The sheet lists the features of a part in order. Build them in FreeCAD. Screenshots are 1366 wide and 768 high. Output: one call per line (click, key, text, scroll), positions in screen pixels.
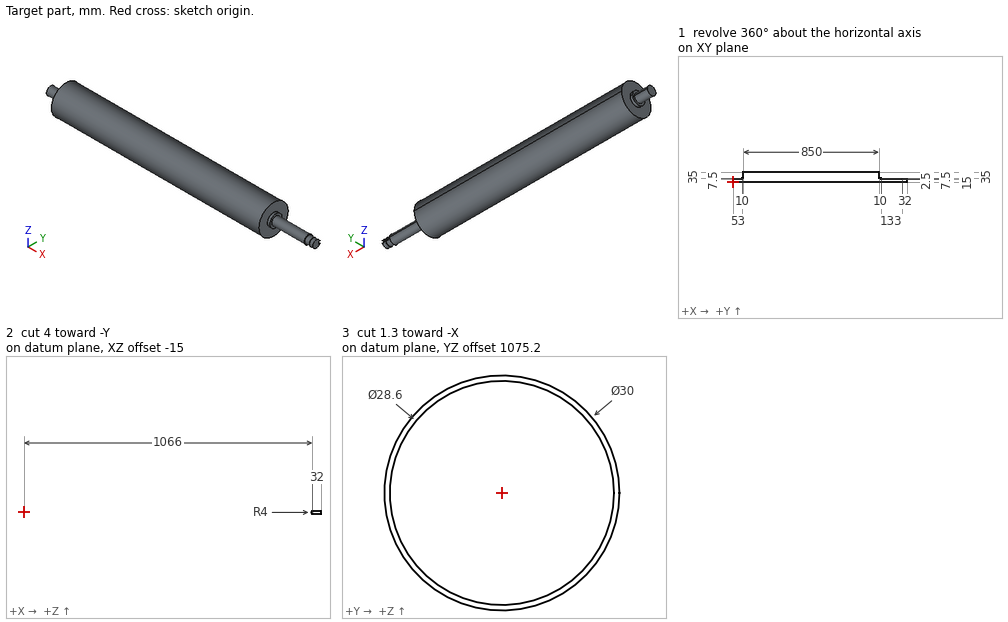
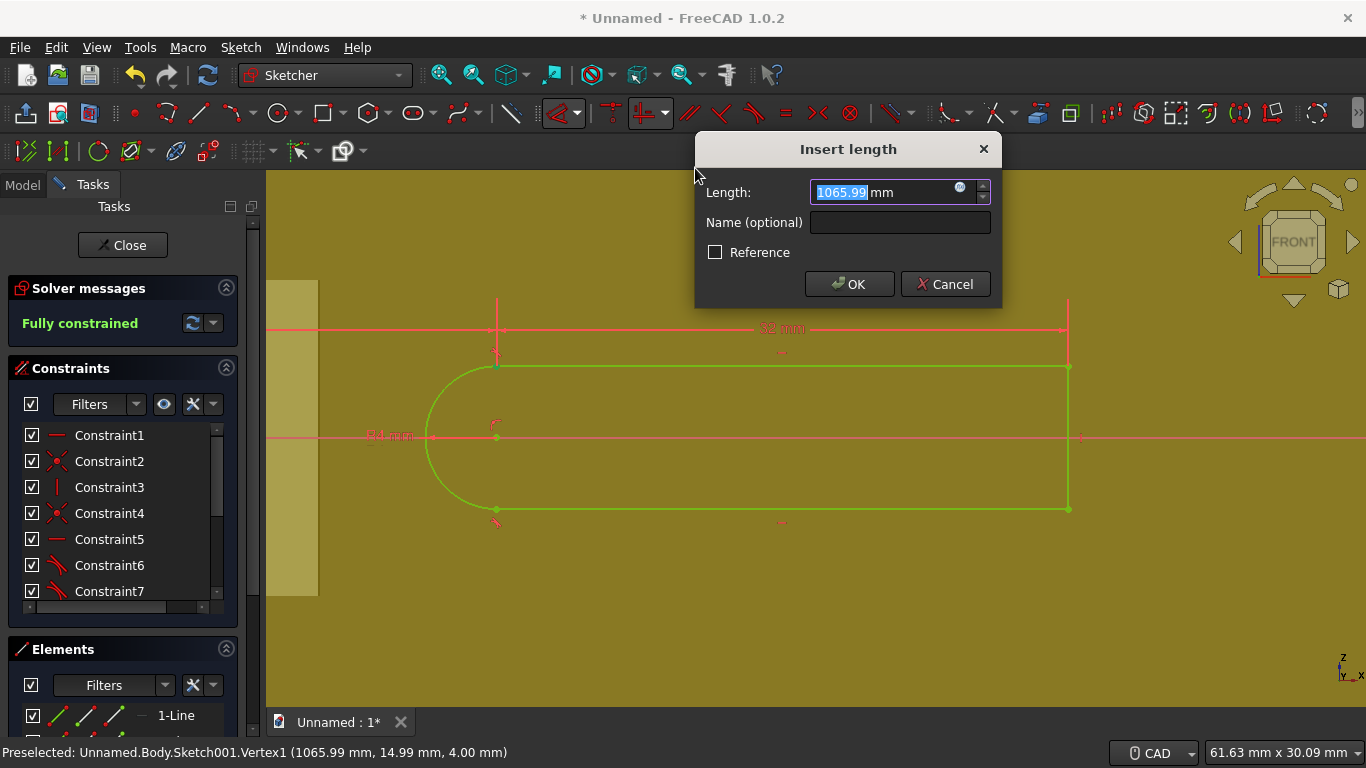
text(1066)
key(Return)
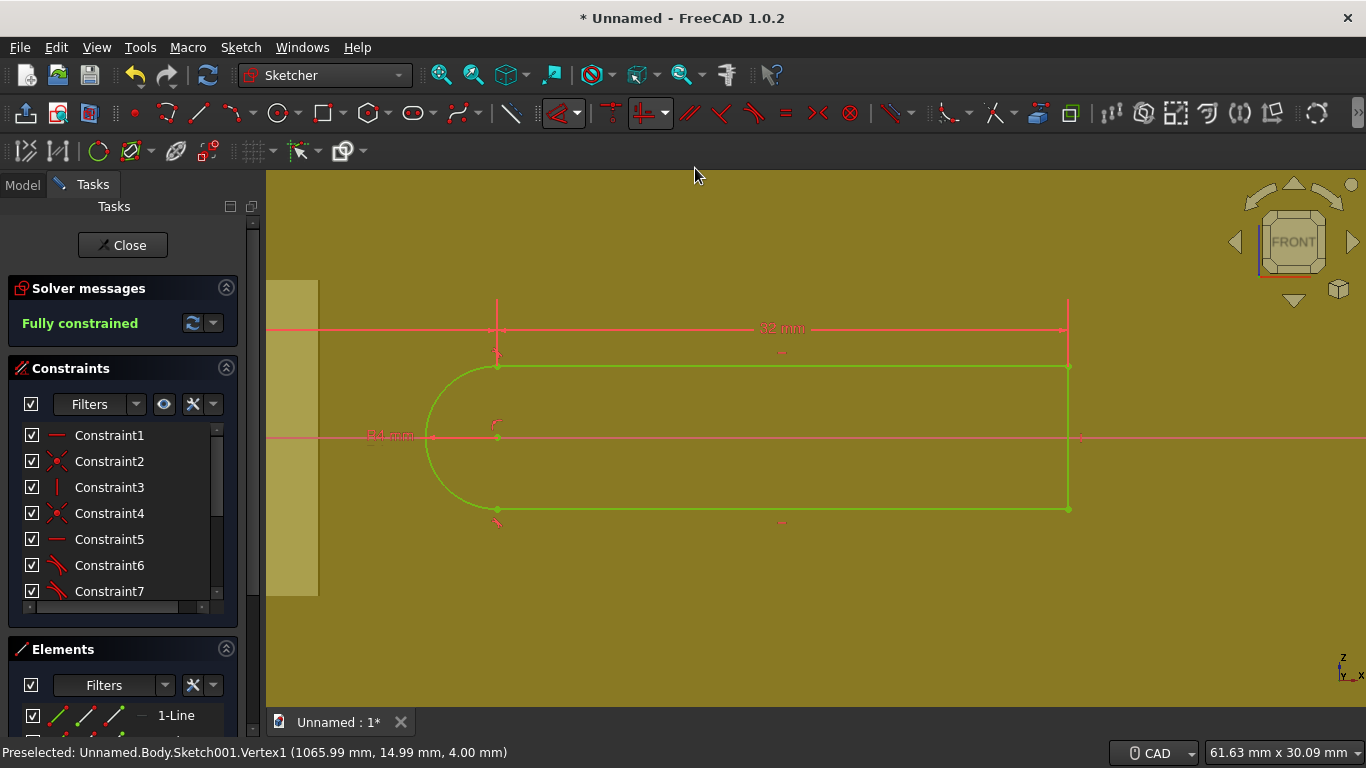
click(123, 245)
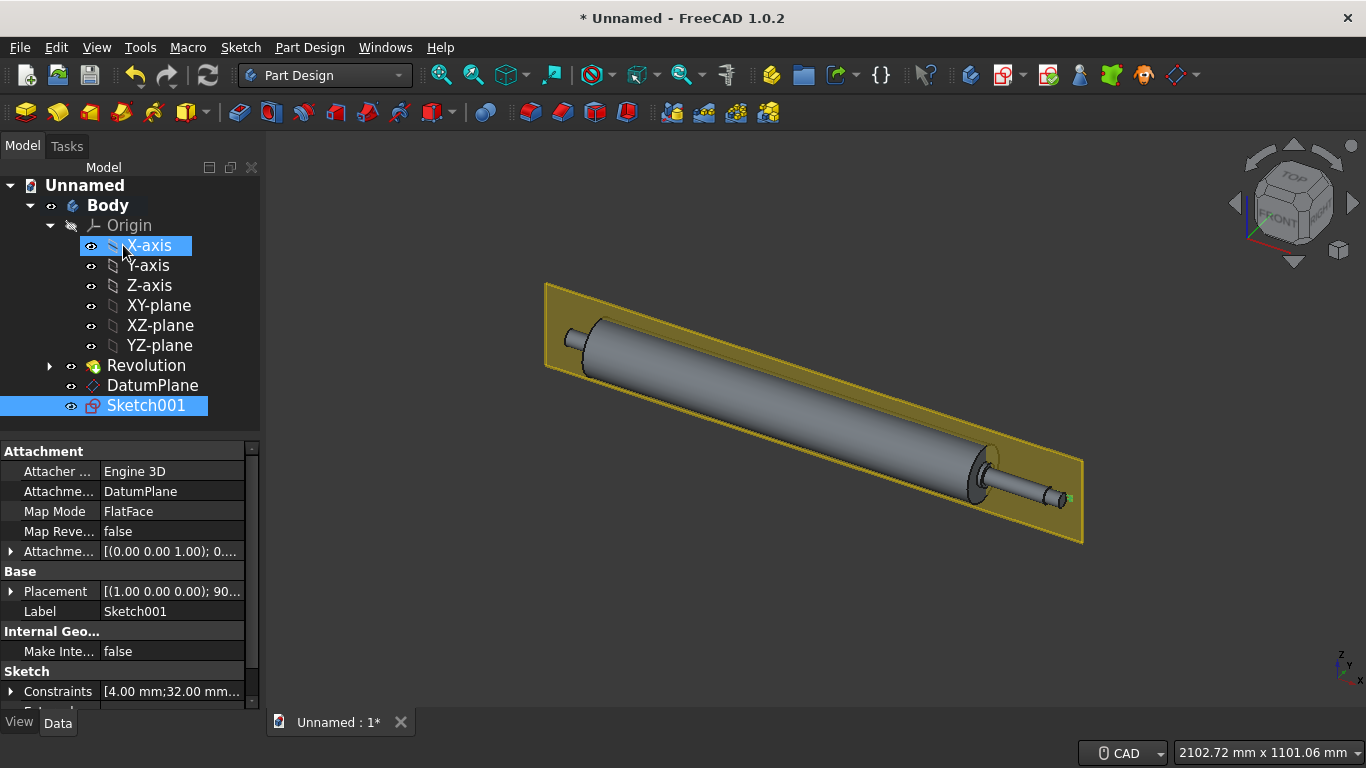
click(240, 112)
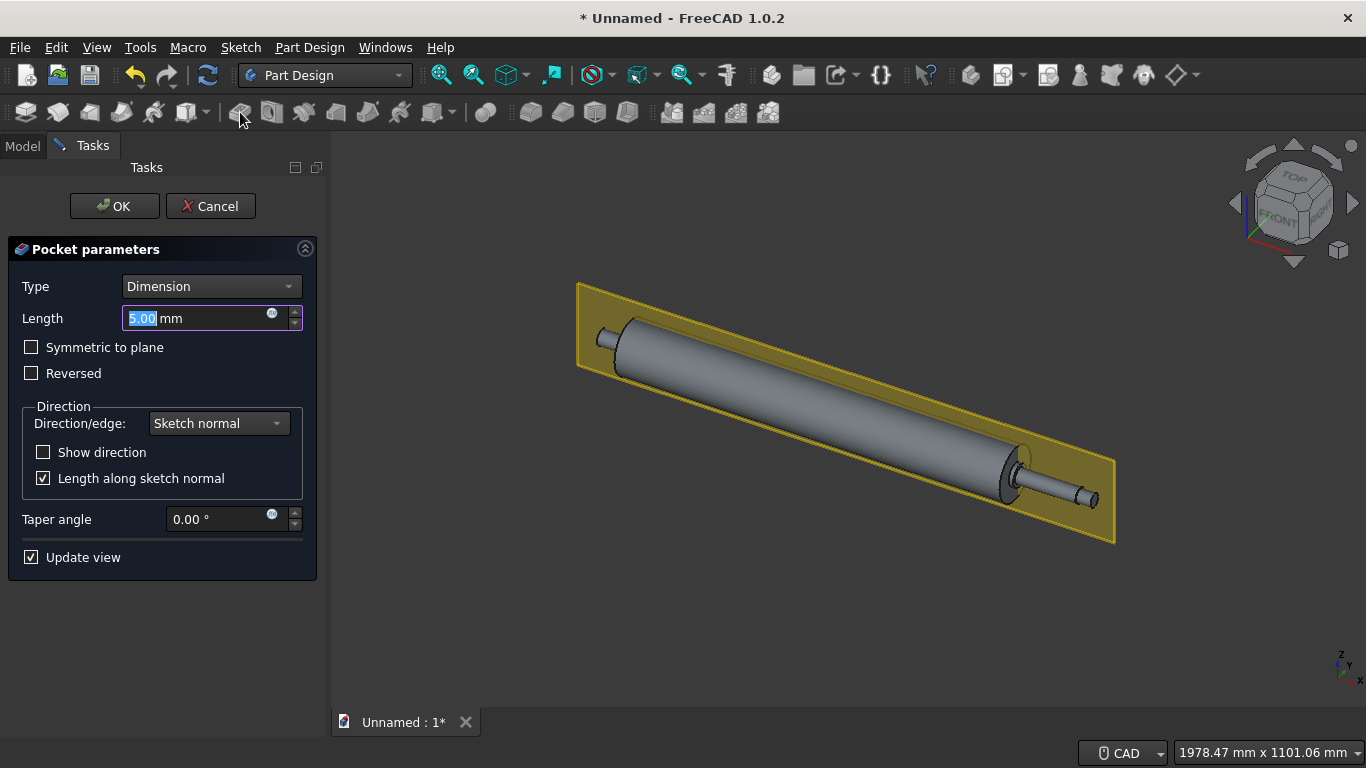
text(4)
key(Tab)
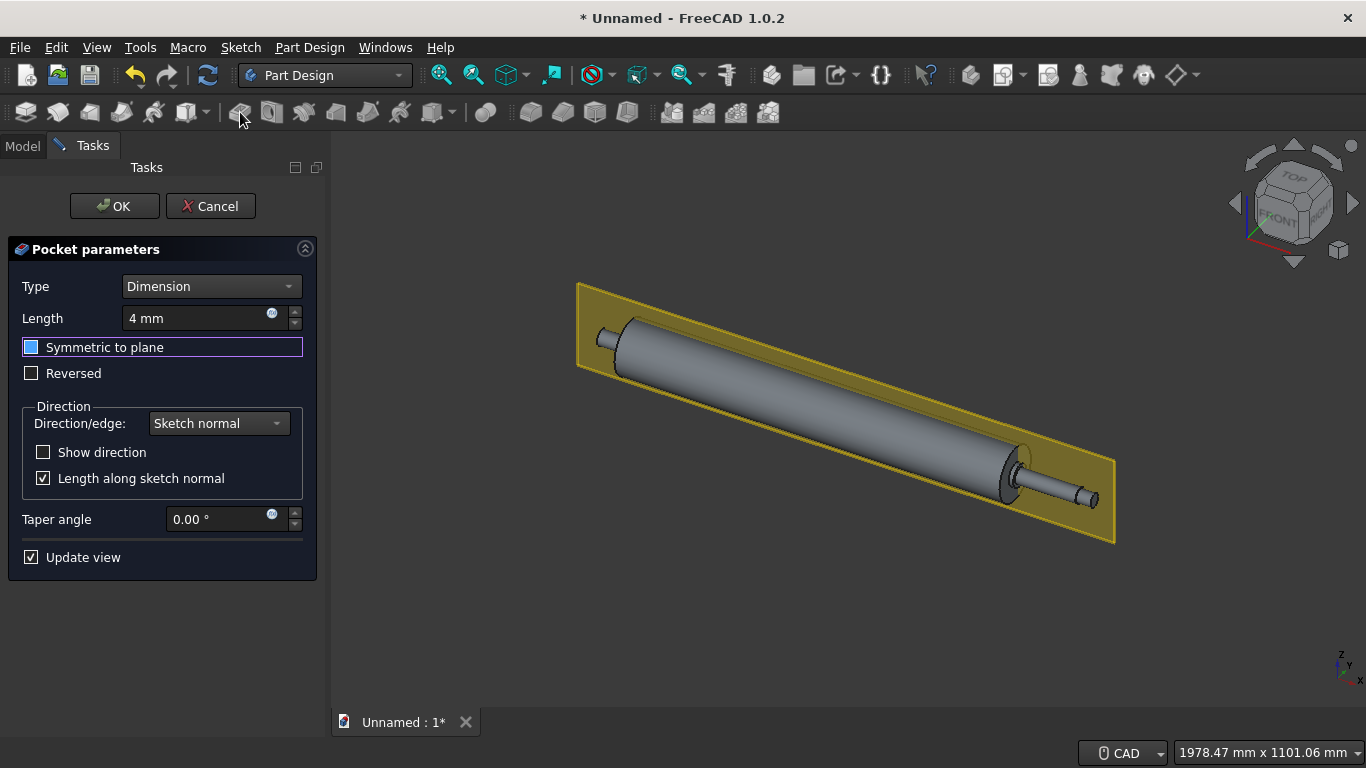
click(30, 373)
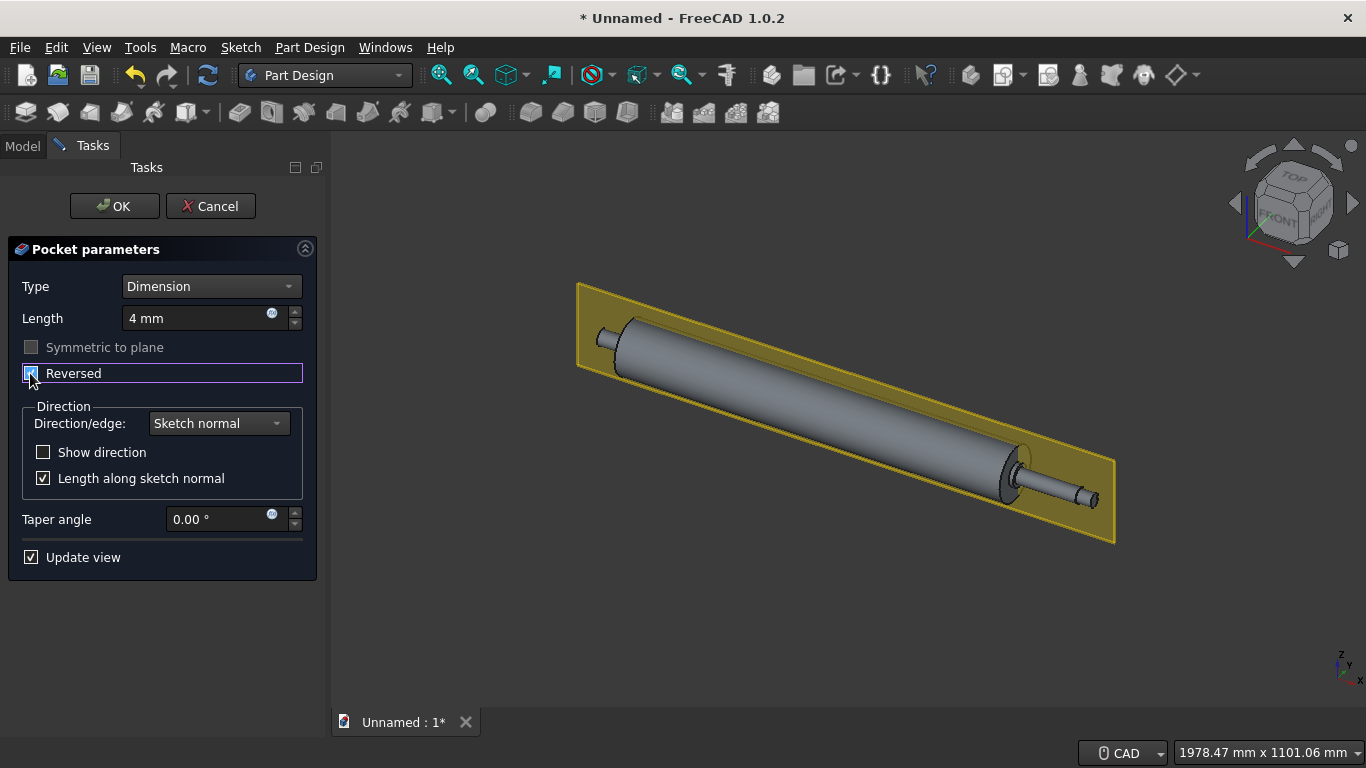
click(115, 206)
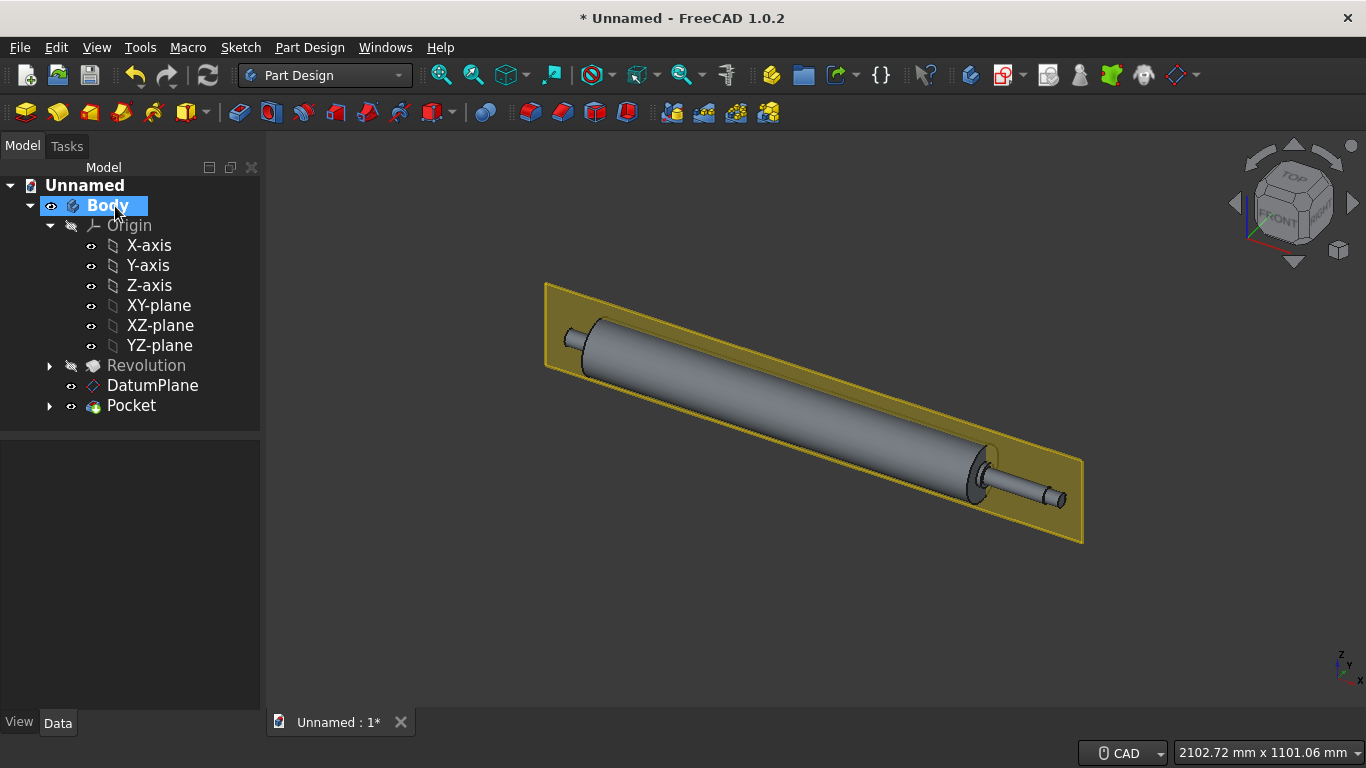
click(116, 386)
key(space)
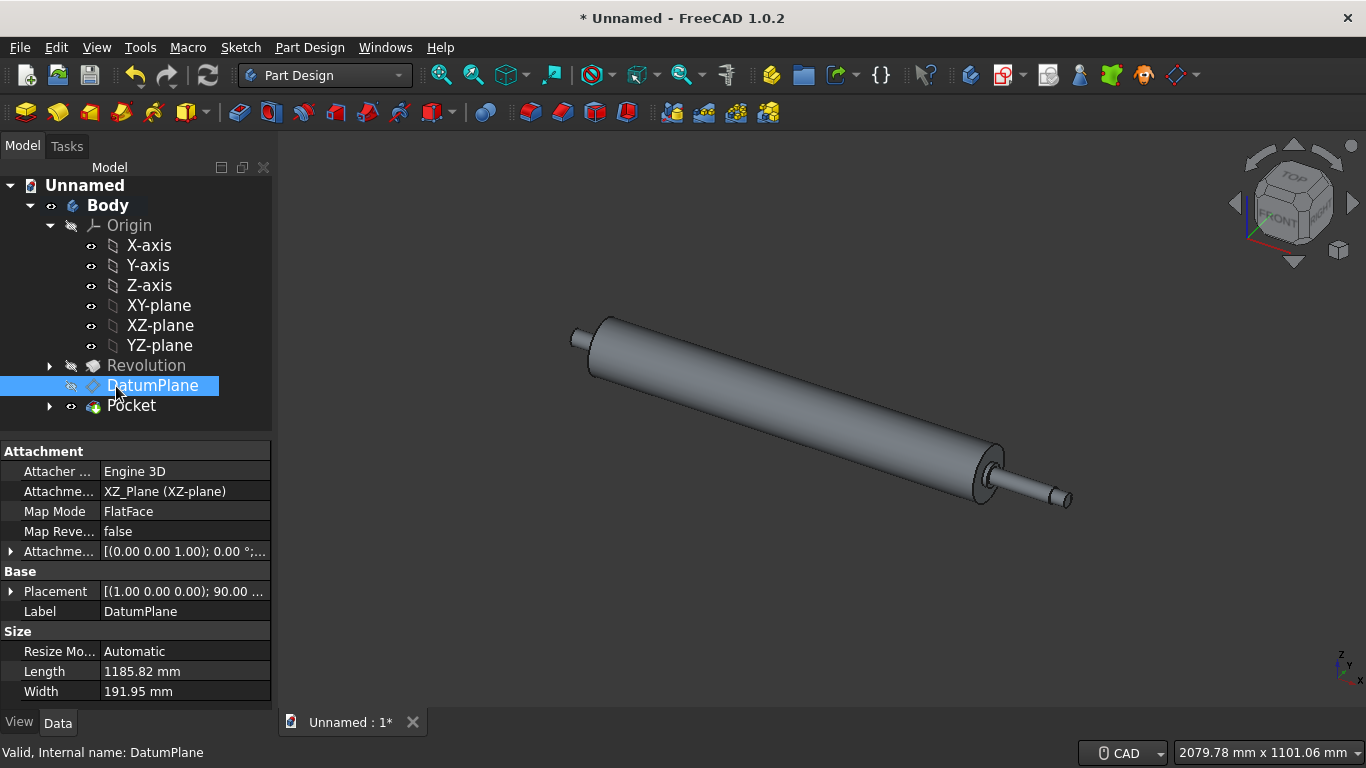
click(136, 346)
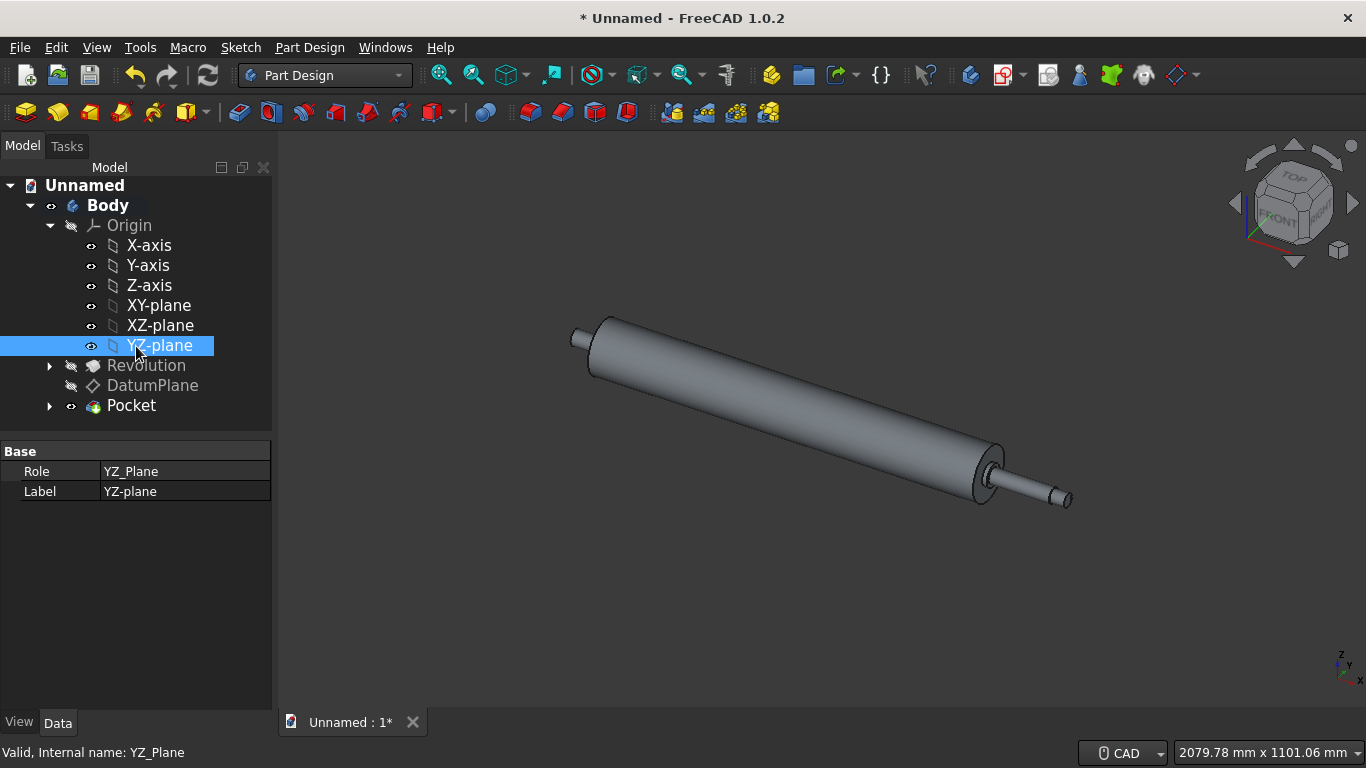
click(1176, 76)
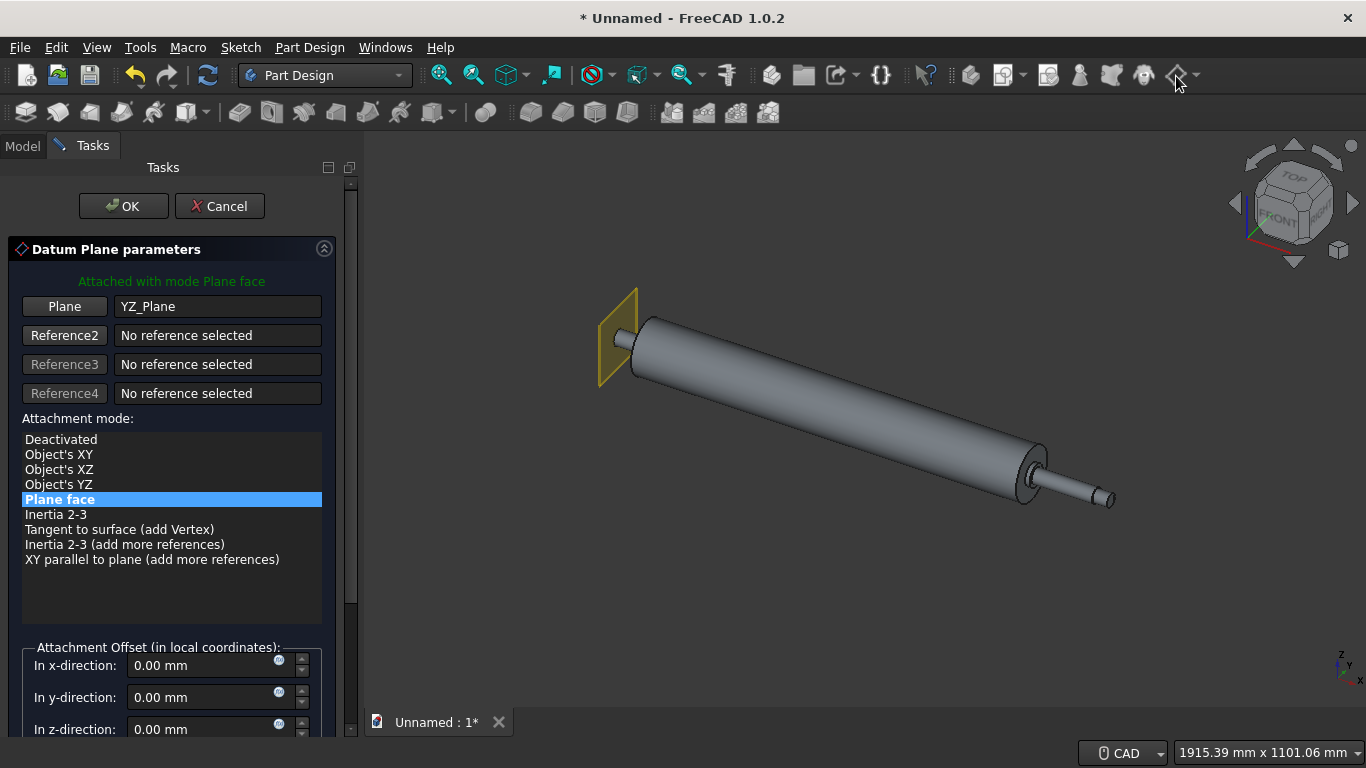
scroll(351, 456, down, 2)